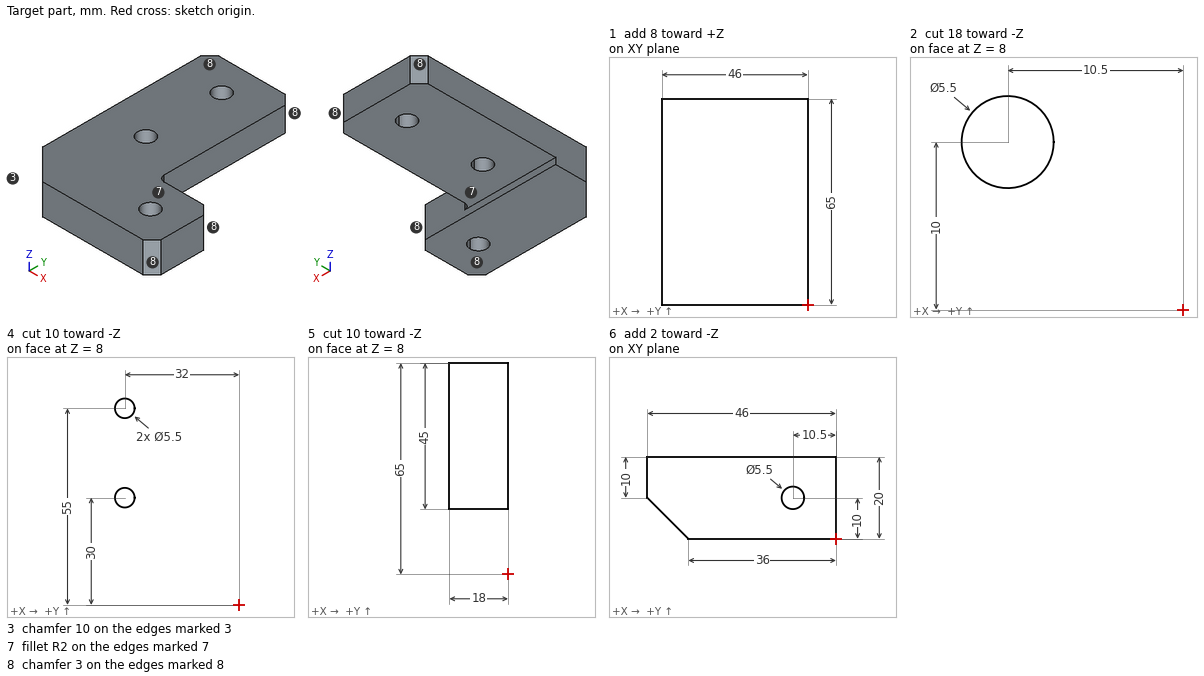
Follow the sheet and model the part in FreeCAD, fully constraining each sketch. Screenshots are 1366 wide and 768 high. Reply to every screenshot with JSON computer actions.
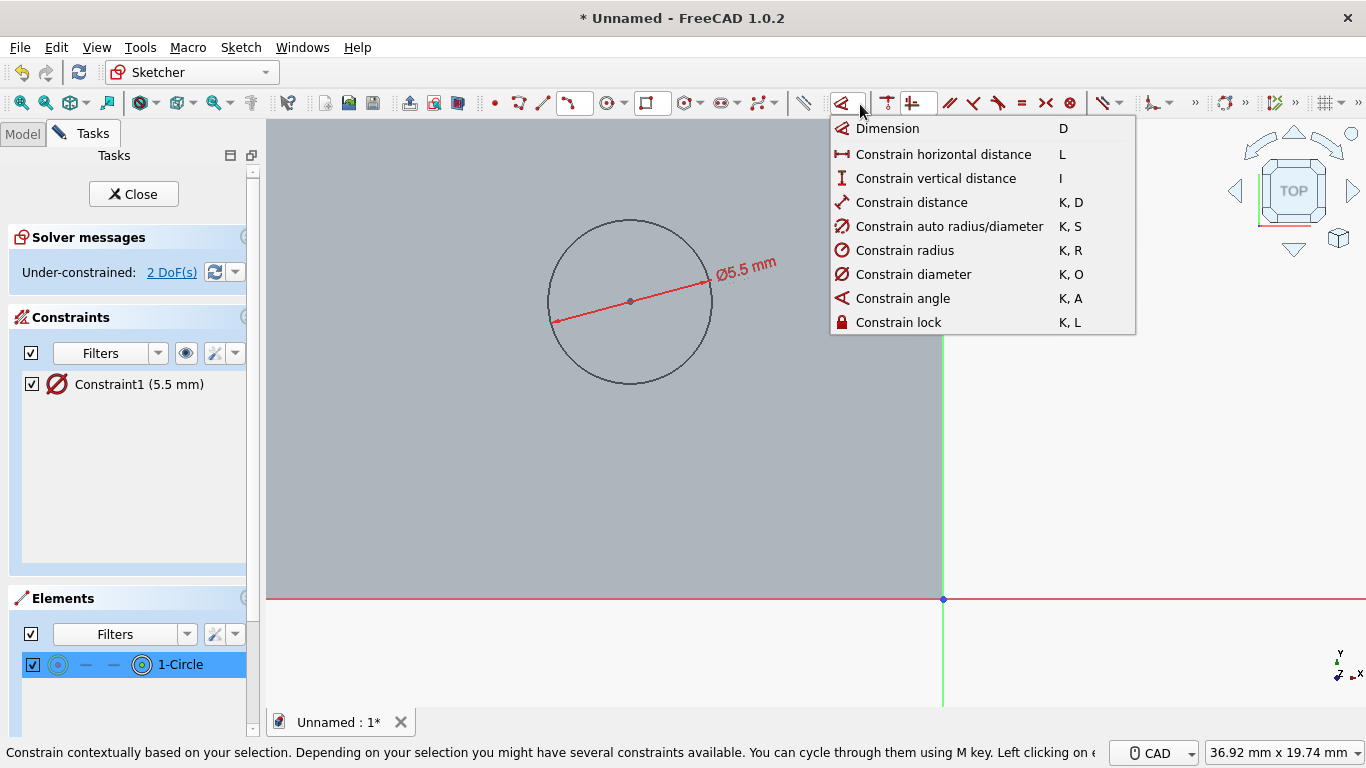
{"action": "left_click", "coordinate": [983, 178]}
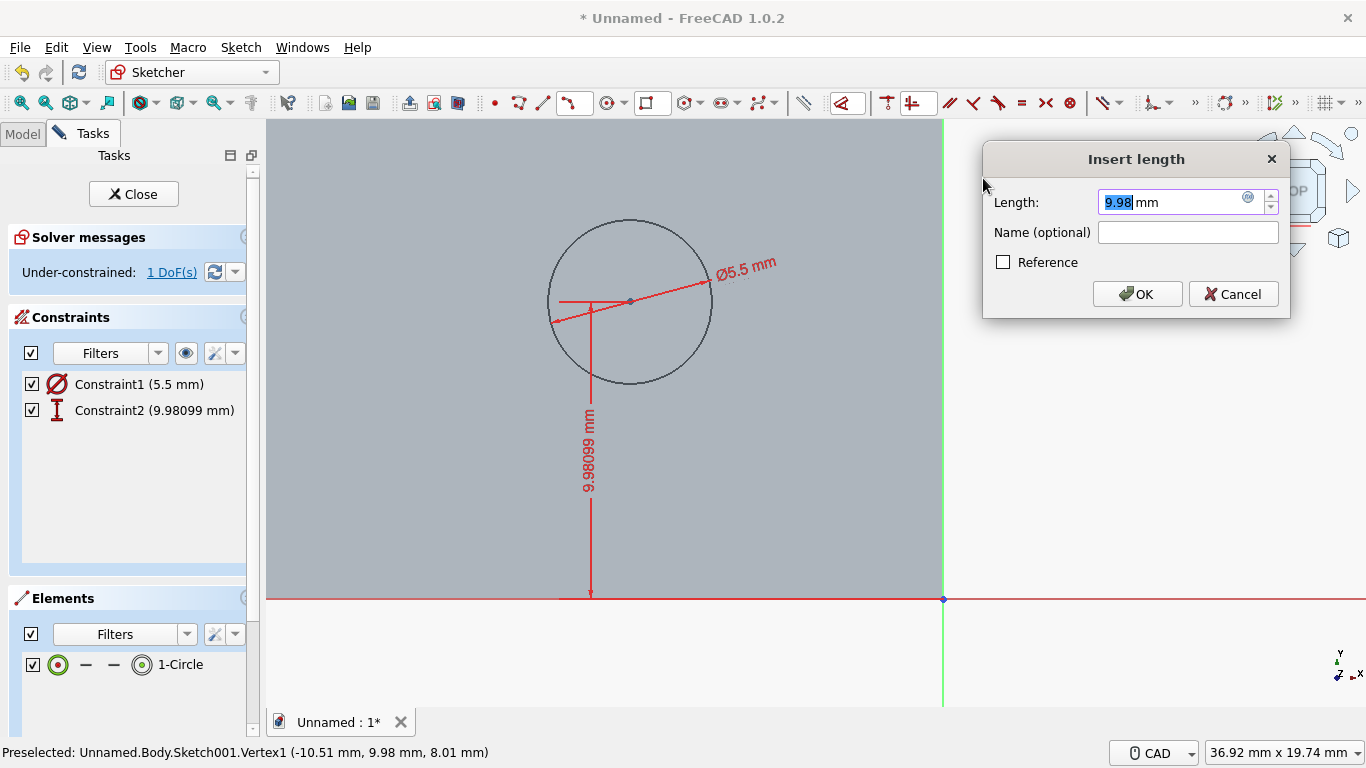
{"action": "type", "text": "10"}
{"action": "key", "text": "Return"}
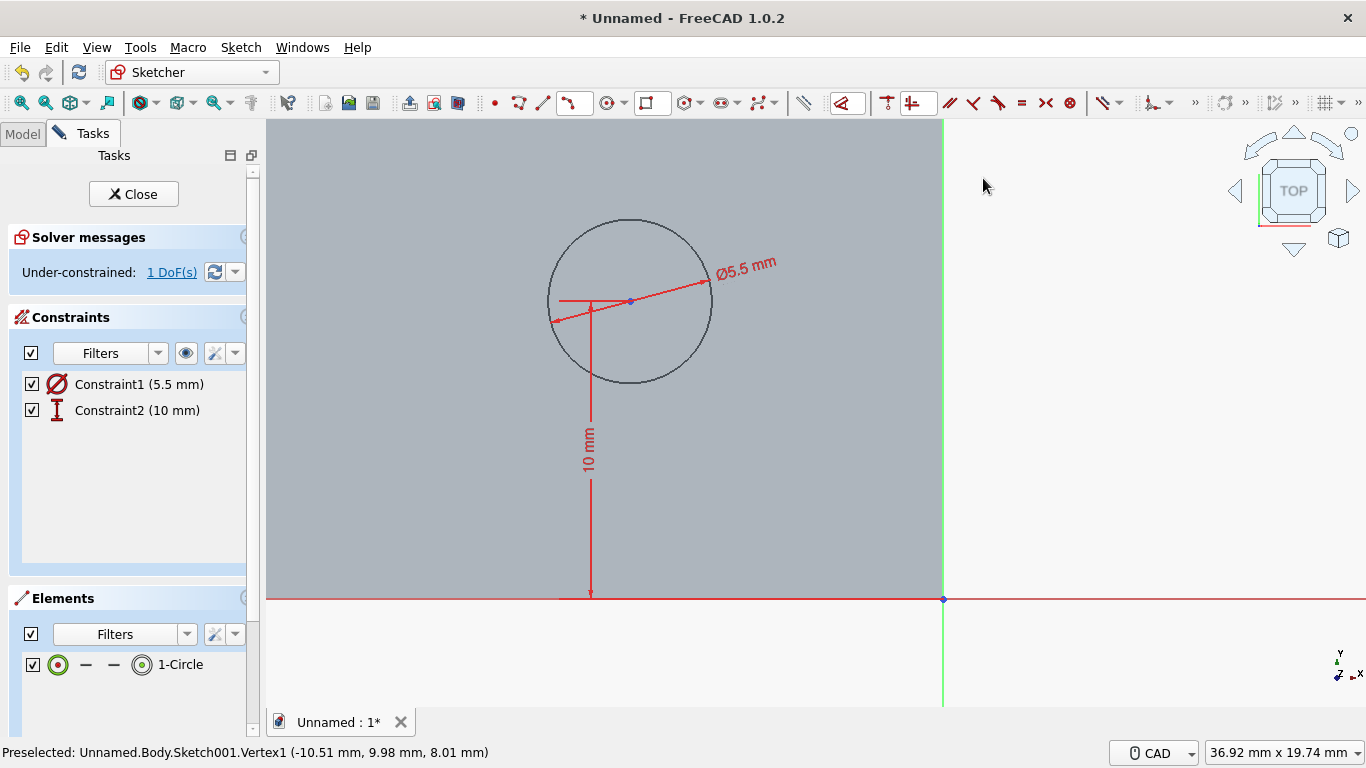
{"action": "left_click", "coordinate": [630, 301]}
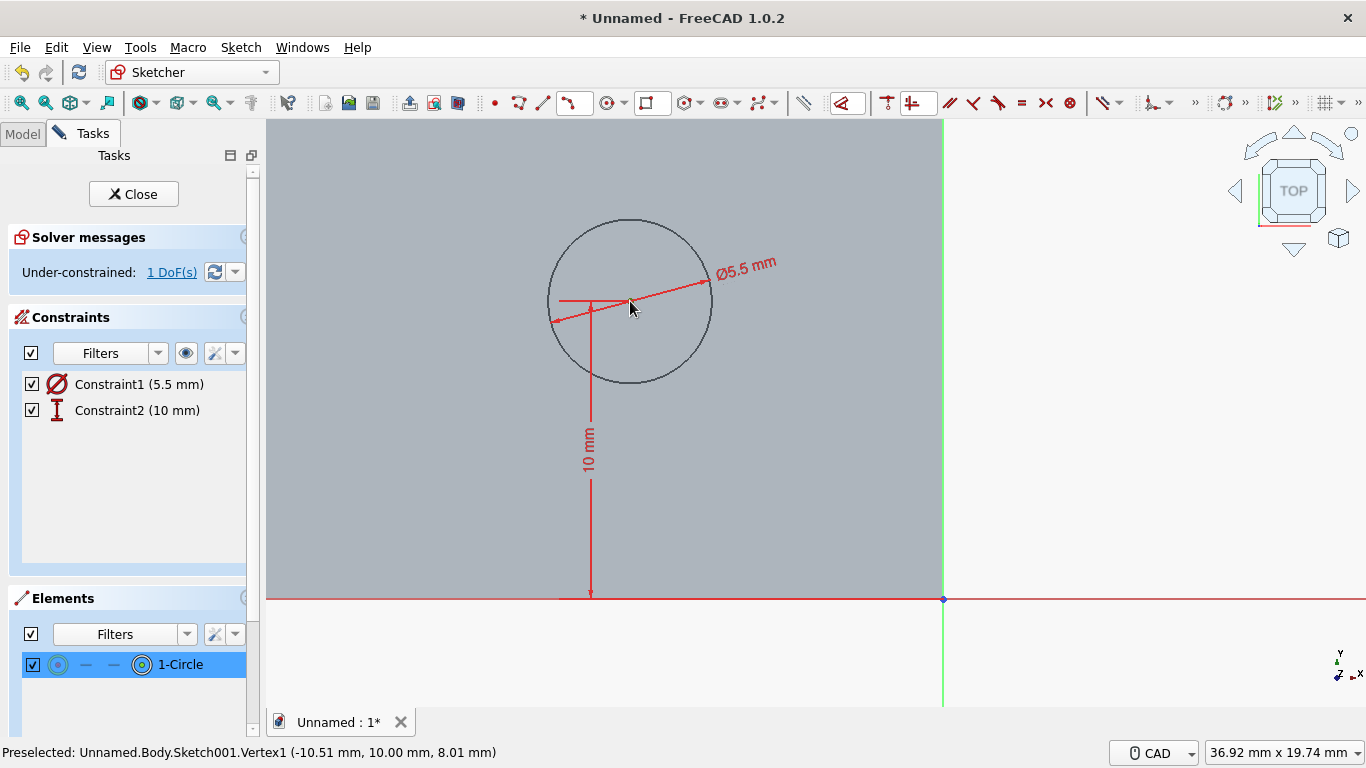
{"action": "left_click", "coordinate": [860, 104]}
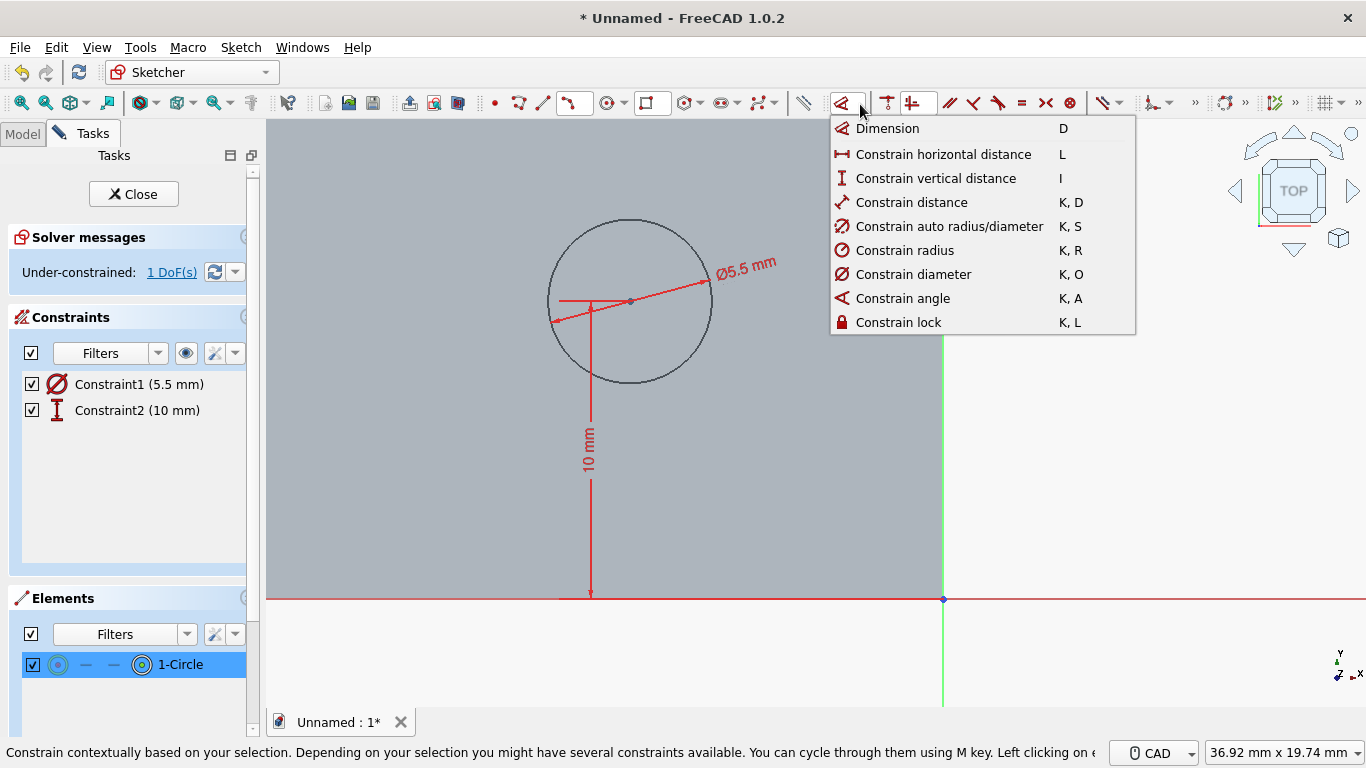
{"action": "left_click", "coordinate": [983, 154]}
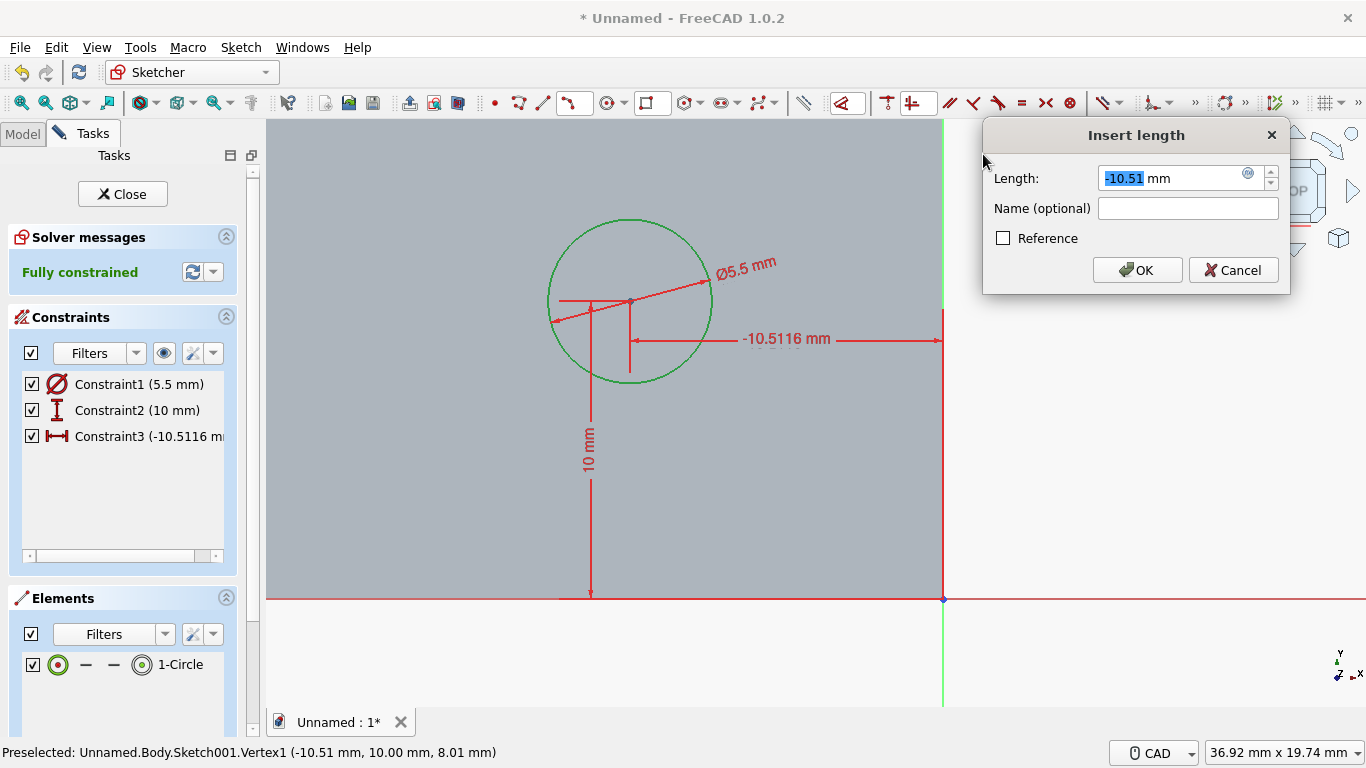
{"action": "type", "text": "-10.5"}
{"action": "key", "text": "Return"}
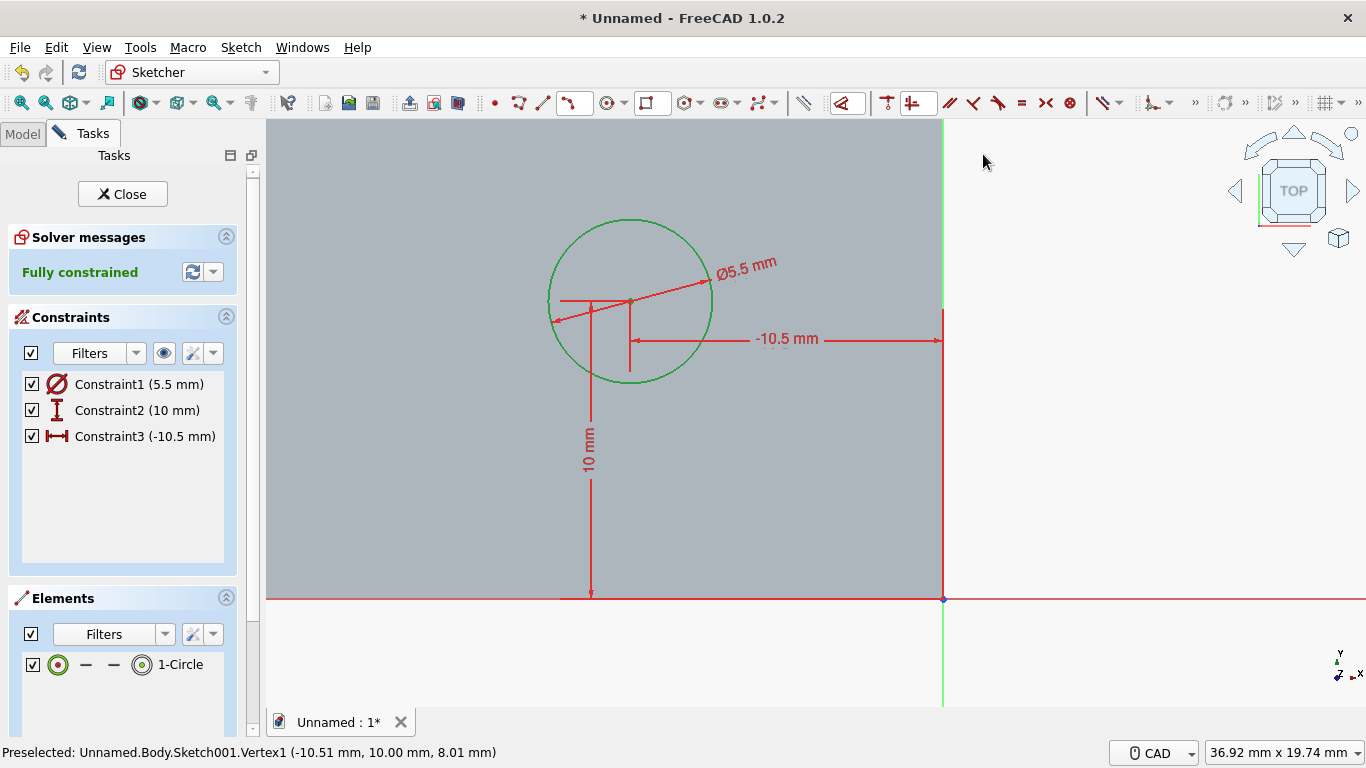
{"action": "left_click", "coordinate": [123, 194]}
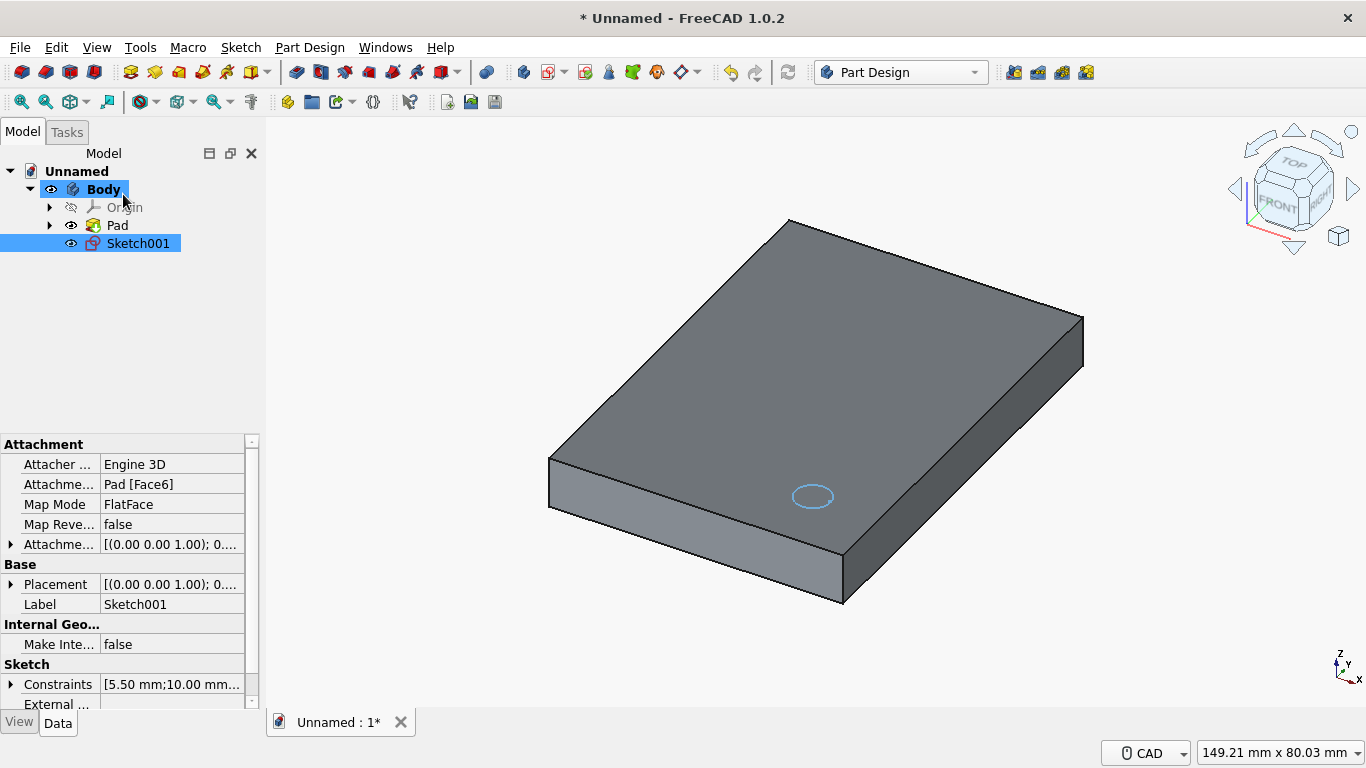
{"action": "left_click", "coordinate": [298, 72]}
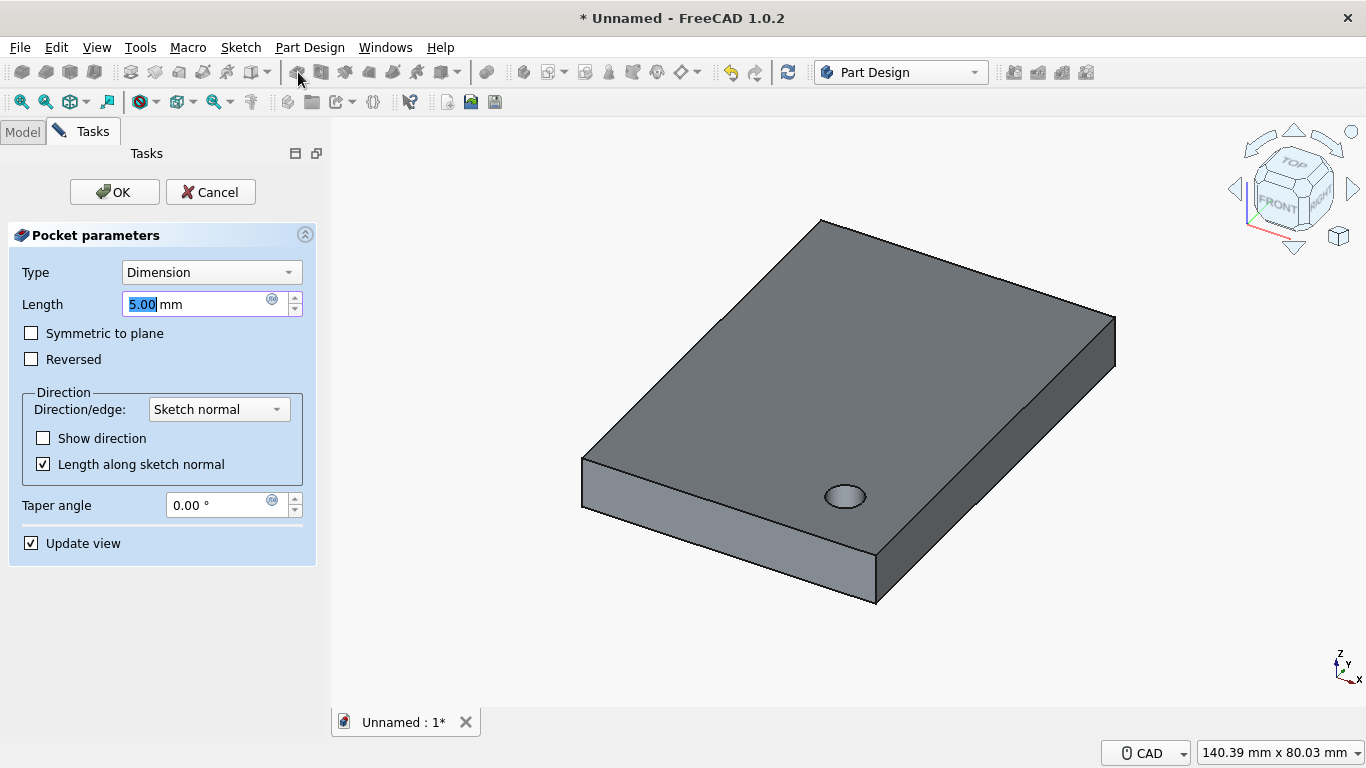
{"action": "type", "text": "18"}
{"action": "key", "text": "Tab"}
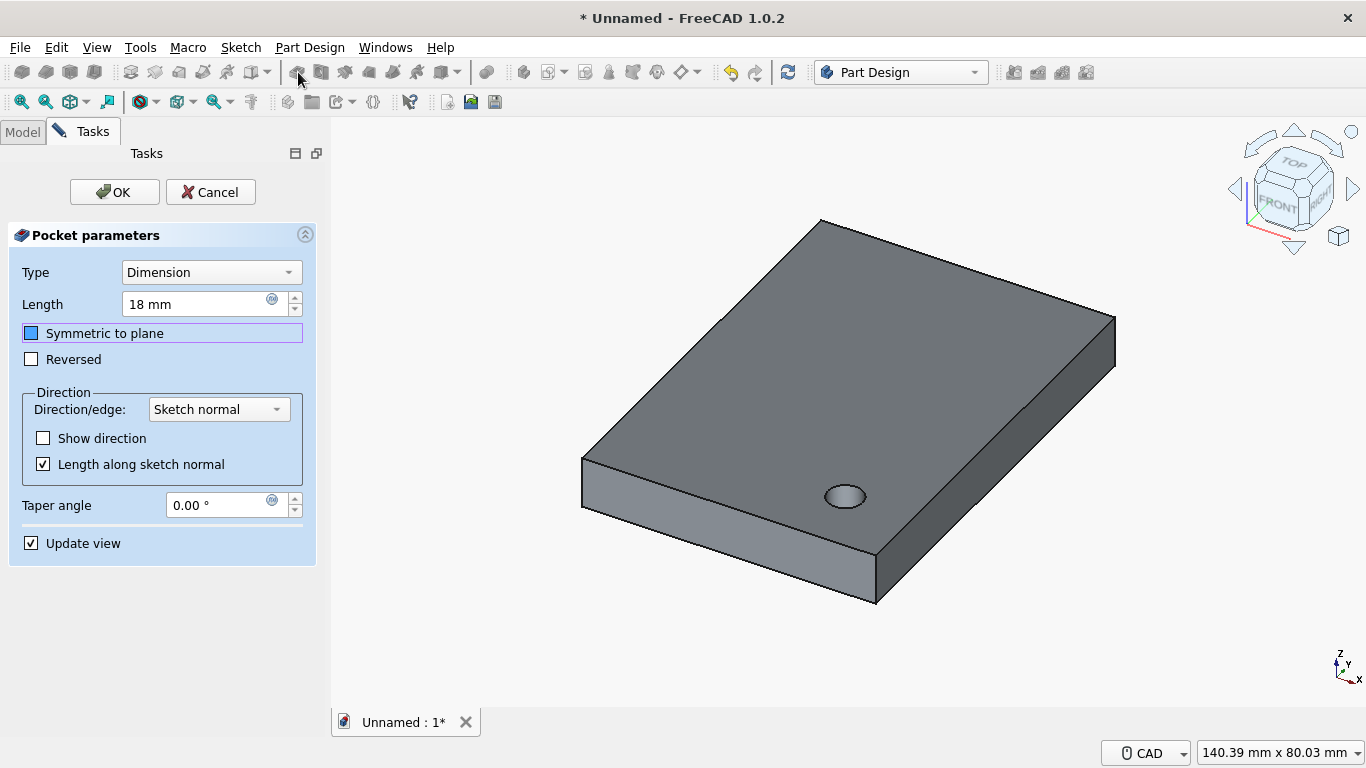
{"action": "left_click", "coordinate": [115, 192]}